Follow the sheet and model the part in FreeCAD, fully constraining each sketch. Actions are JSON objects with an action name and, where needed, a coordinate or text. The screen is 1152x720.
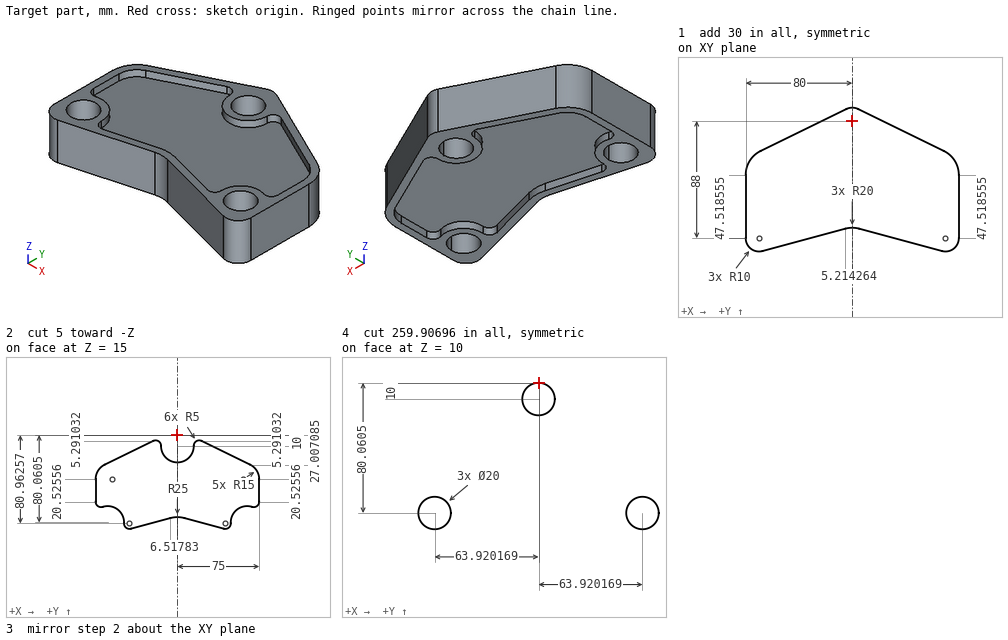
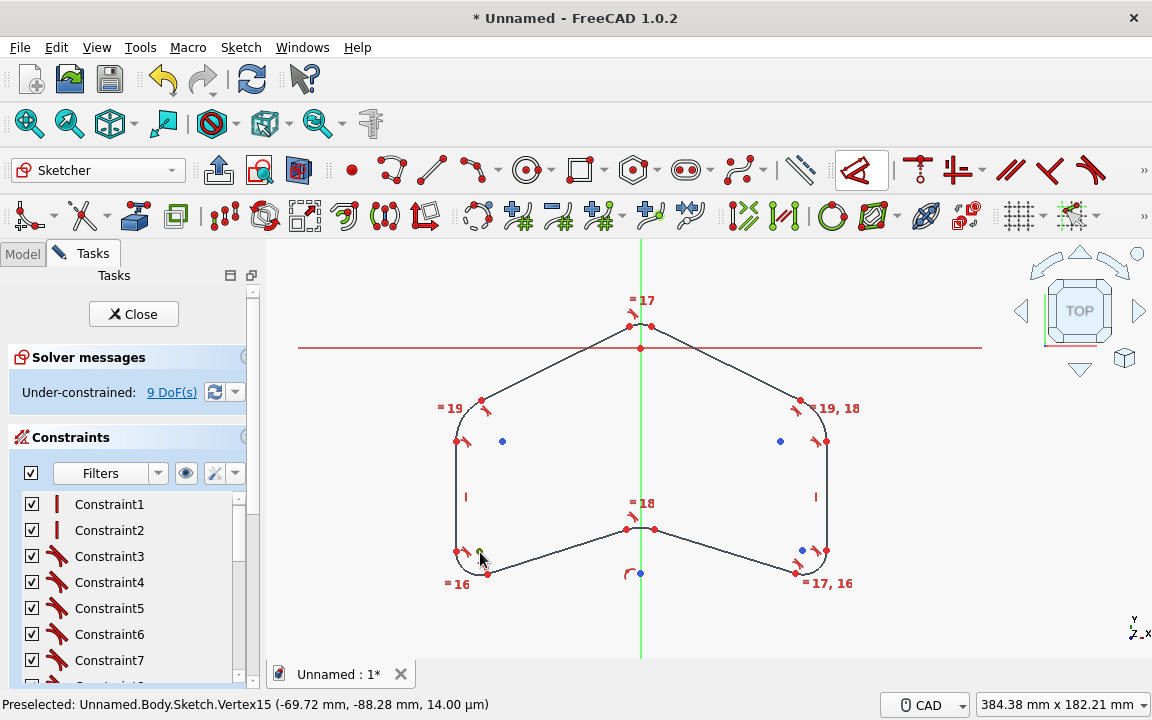
{"action": "left_click", "coordinate": [803, 551]}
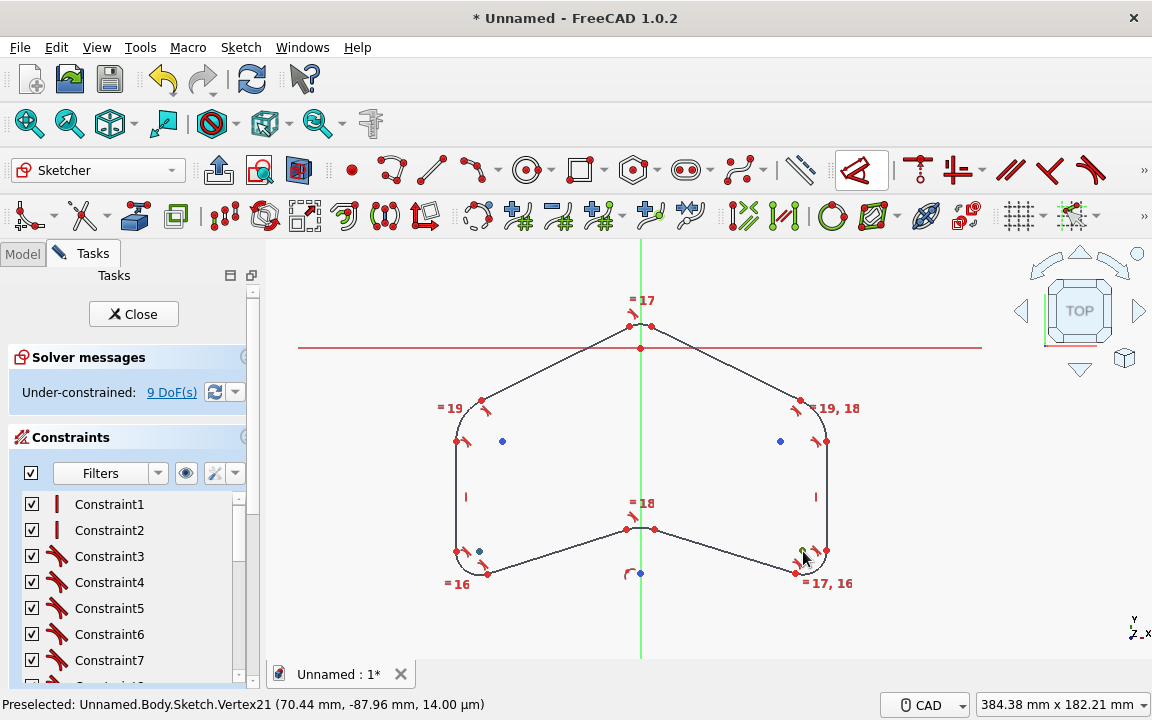
{"action": "left_click", "coordinate": [641, 605]}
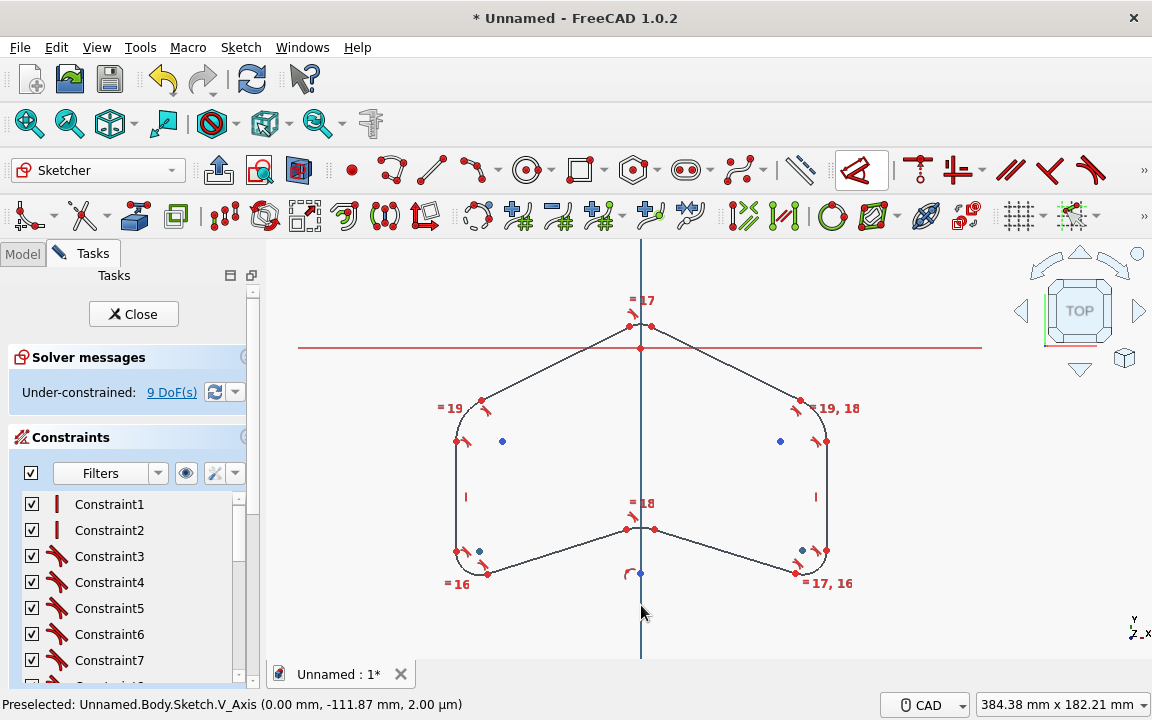
{"action": "key", "text": "s"}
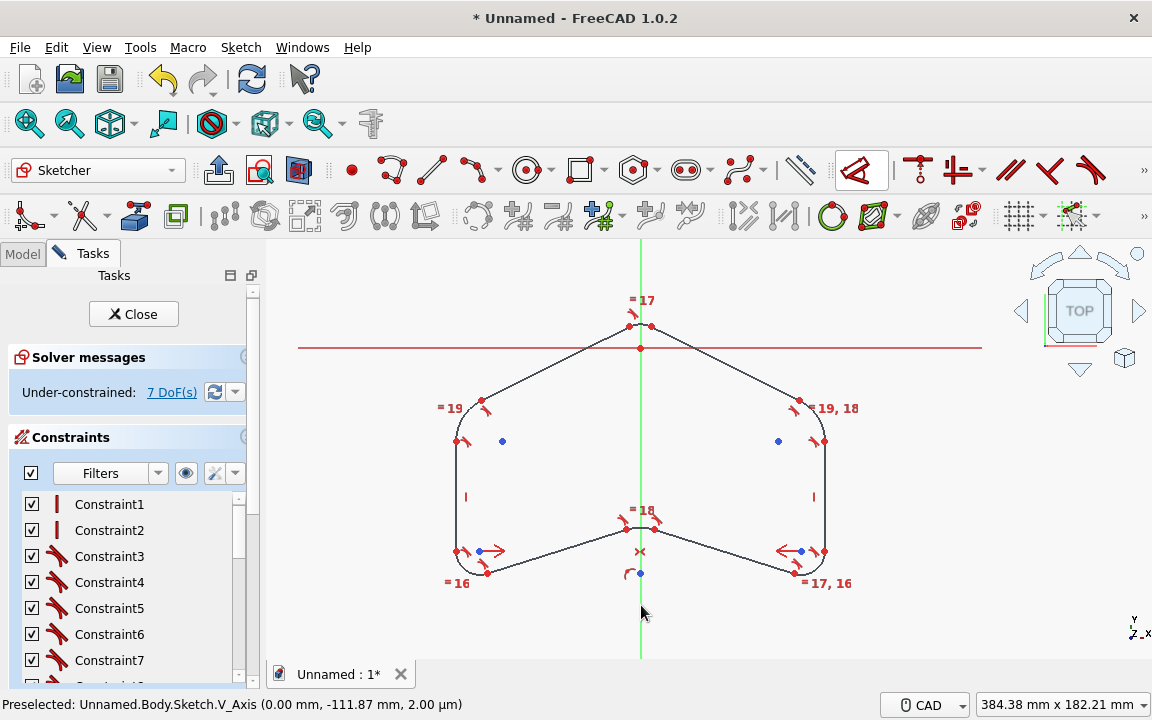
{"action": "scroll", "coordinate": [460, 564], "scroll_direction": "up", "scroll_amount": 3}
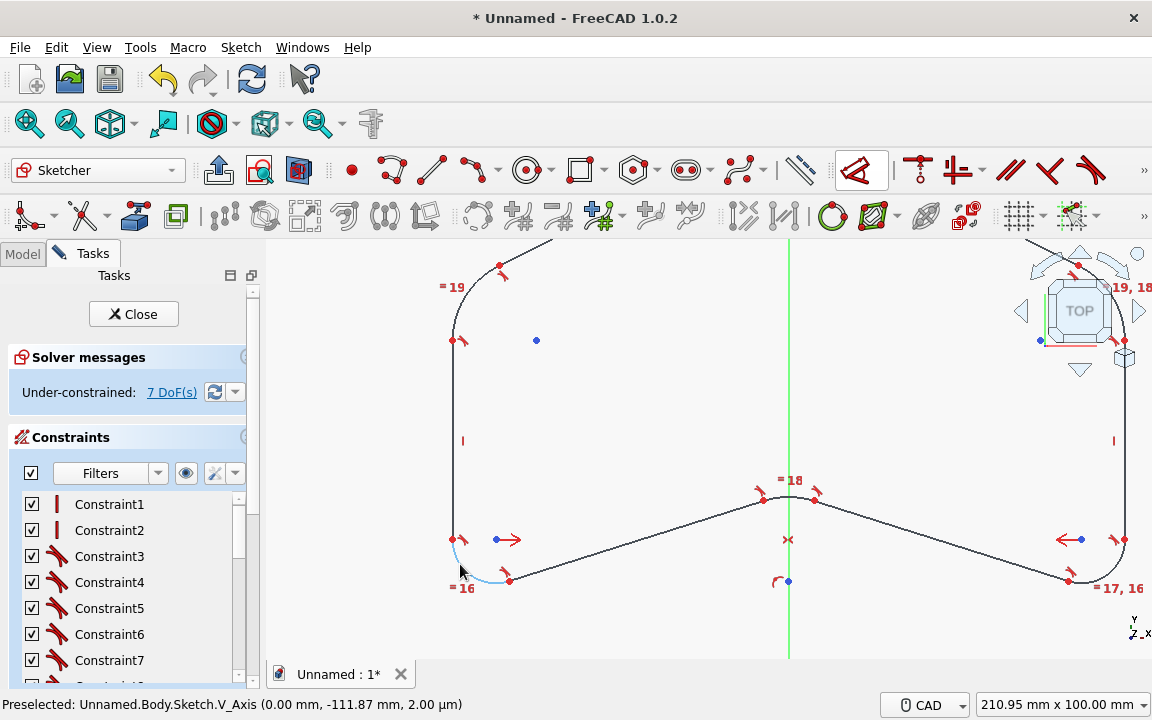
{"action": "left_click", "coordinate": [459, 563]}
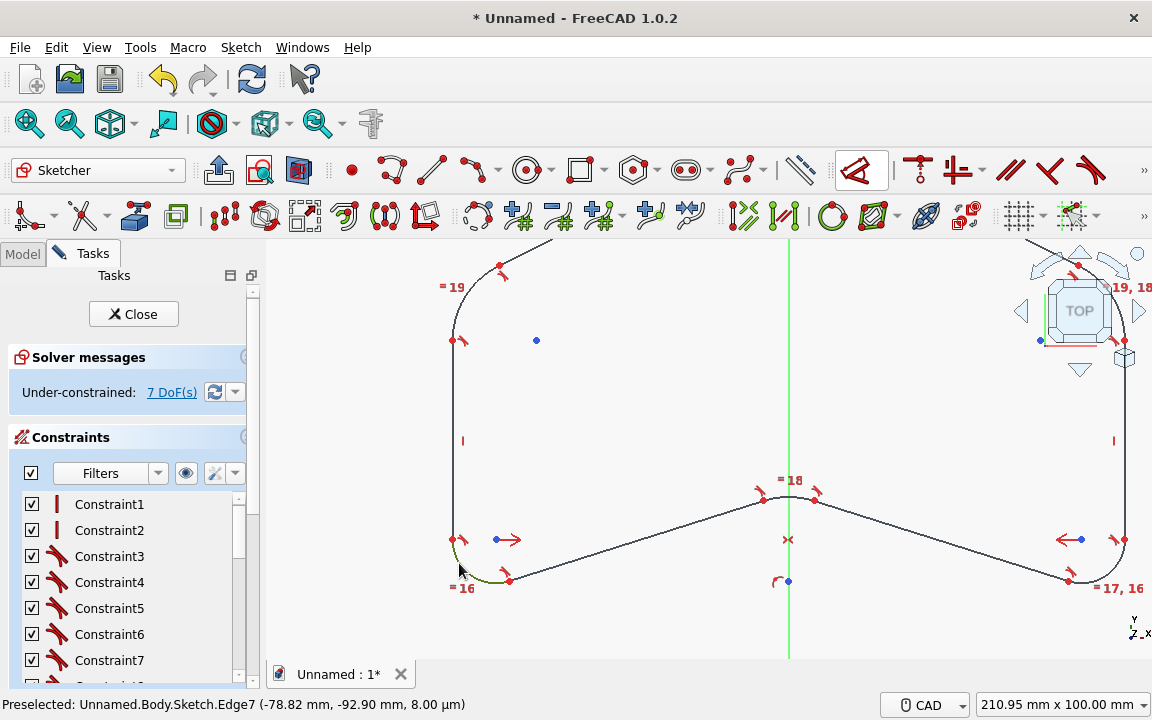
{"action": "key", "text": "k r"}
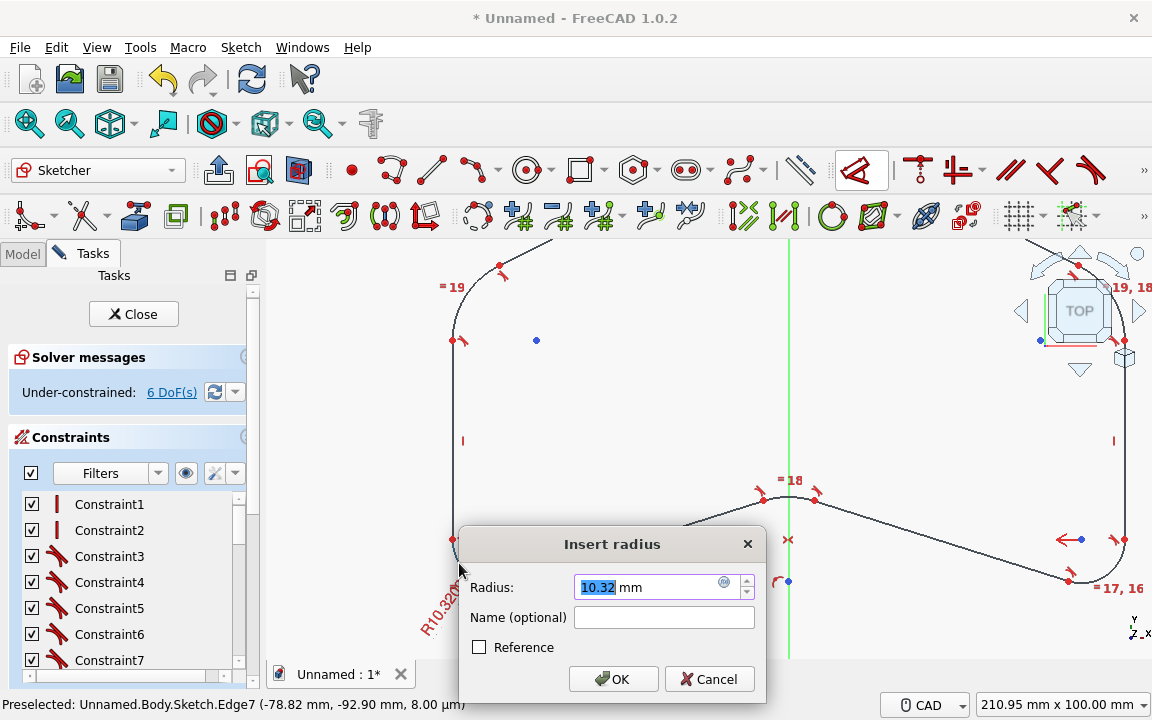
{"action": "type", "text": "10"}
{"action": "key", "text": "Return"}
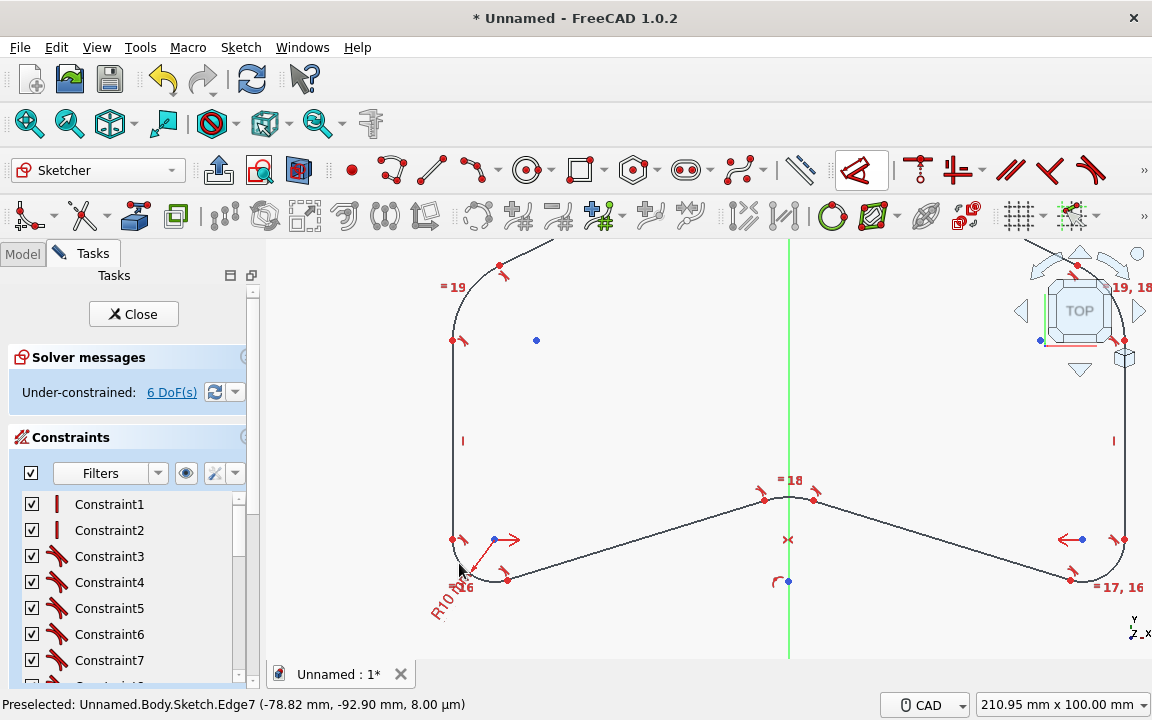
{"action": "scroll", "coordinate": [799, 498], "scroll_direction": "up", "scroll_amount": 2}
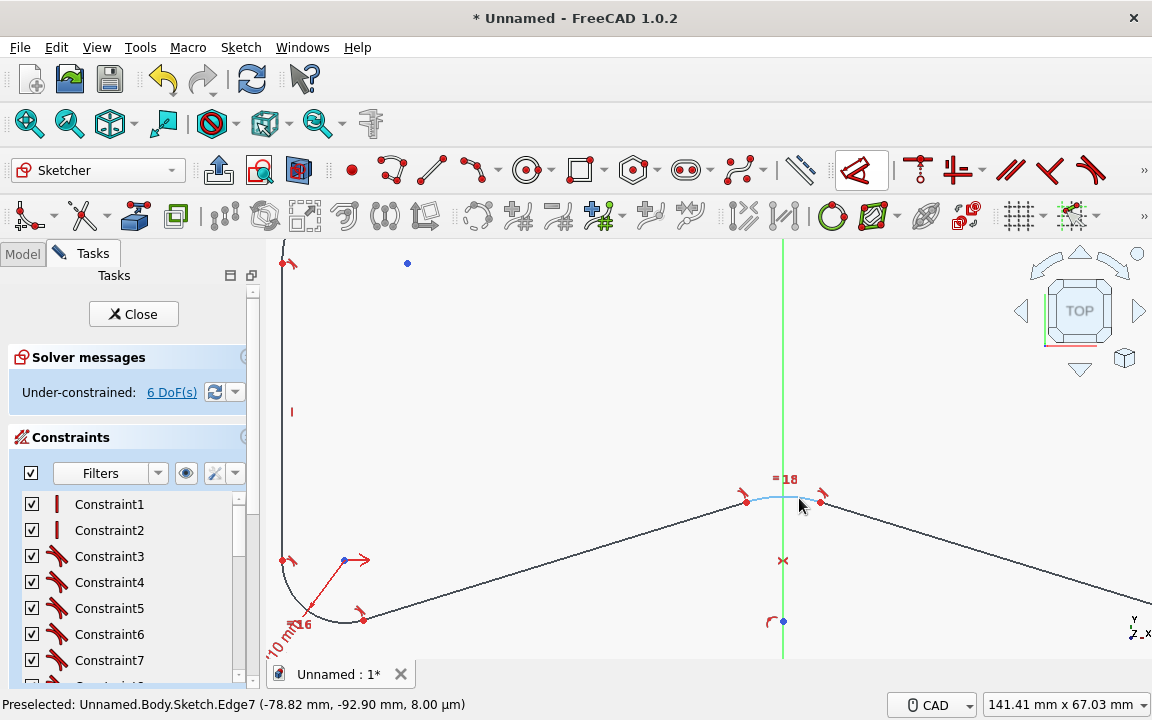
{"action": "left_click", "coordinate": [798, 497]}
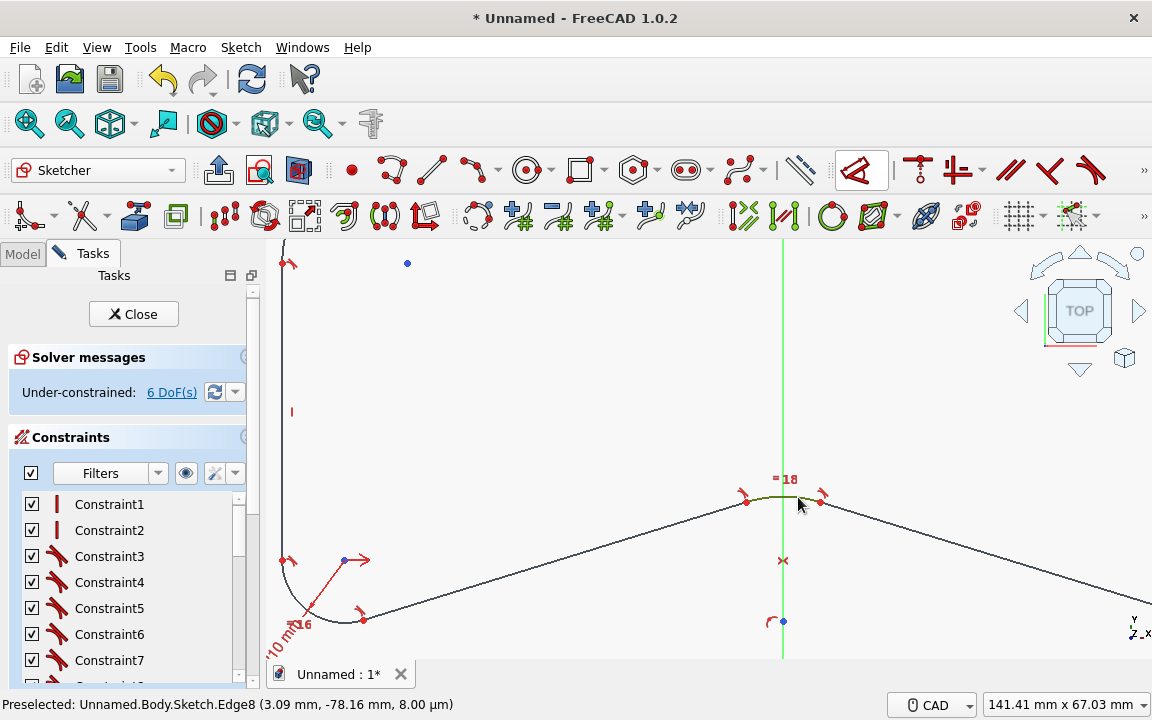
{"action": "key", "text": "k r"}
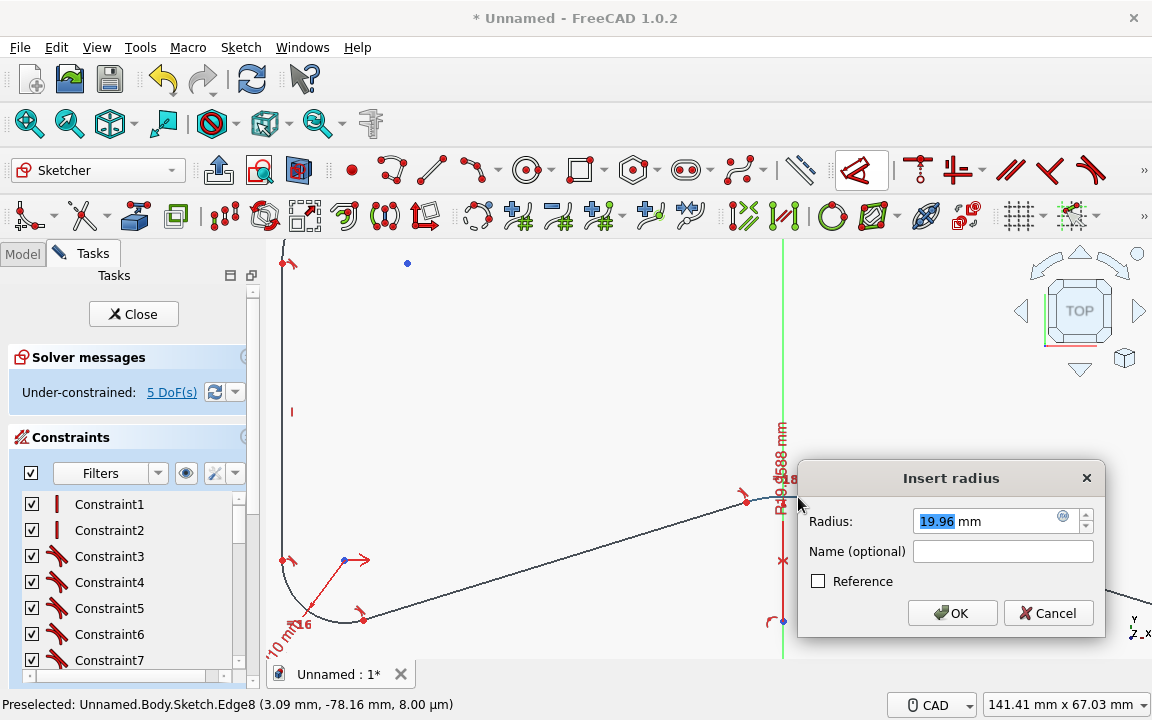
{"action": "type", "text": "20"}
{"action": "key", "text": "Return"}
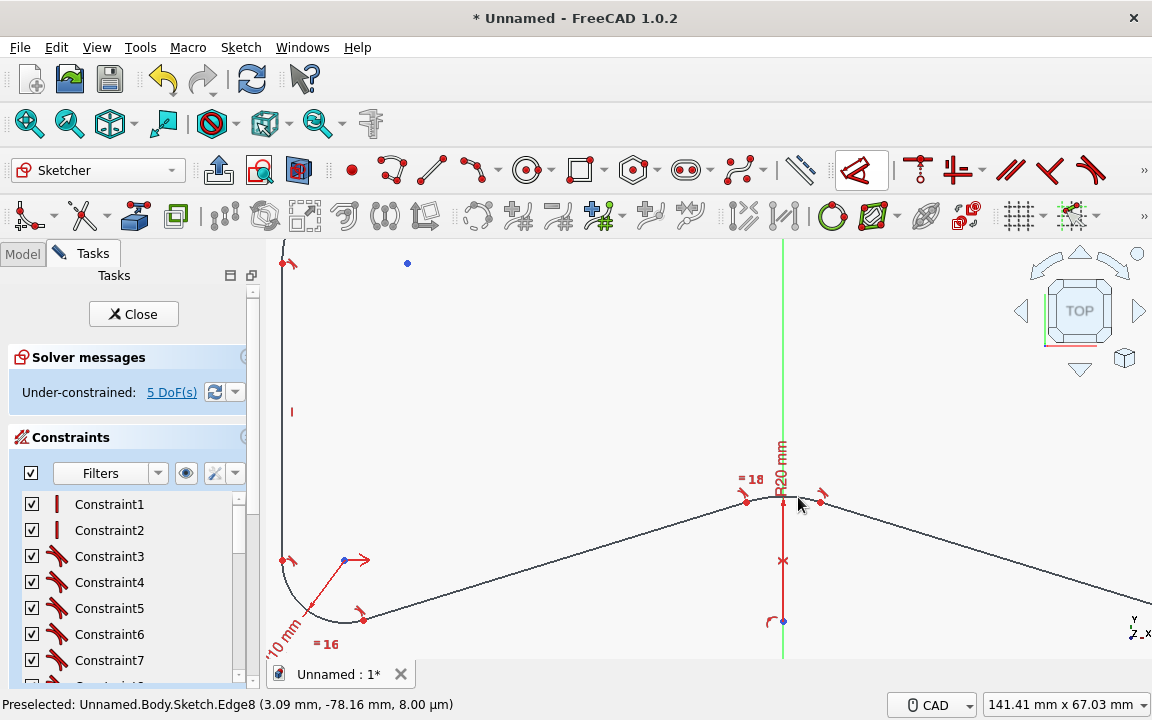
{"action": "scroll", "coordinate": [557, 546], "scroll_direction": "down", "scroll_amount": 5}